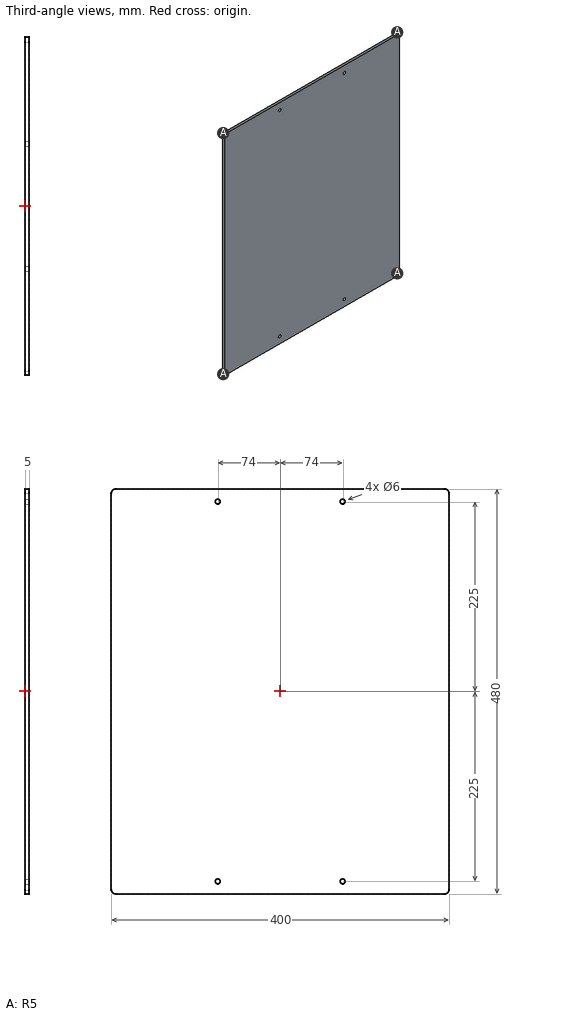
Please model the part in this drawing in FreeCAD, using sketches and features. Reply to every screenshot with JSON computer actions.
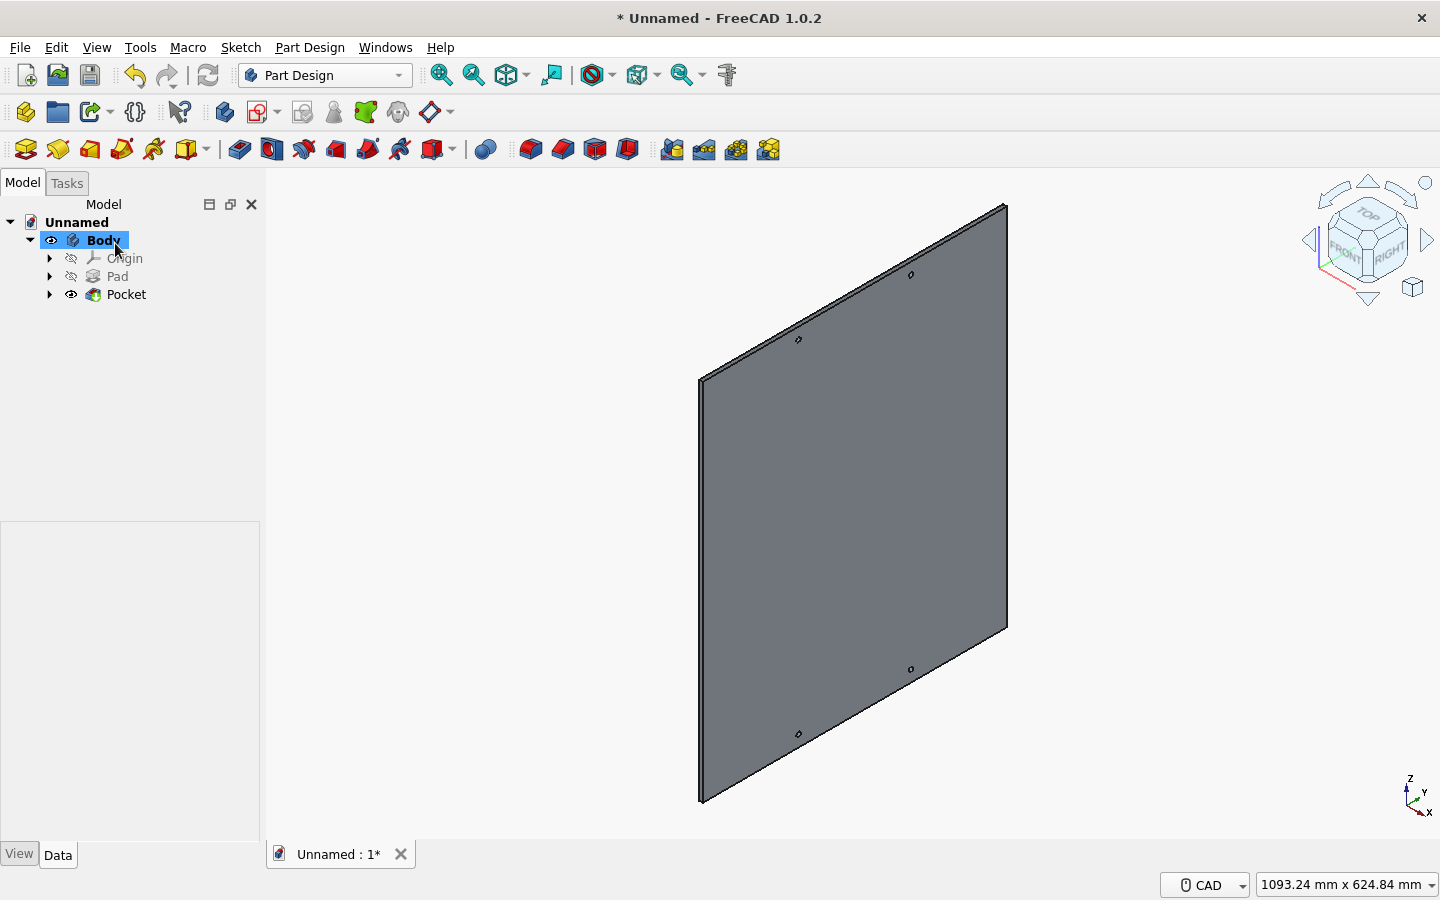
{"action": "scroll", "coordinate": [1005, 204], "scroll_direction": "up", "scroll_amount": 11}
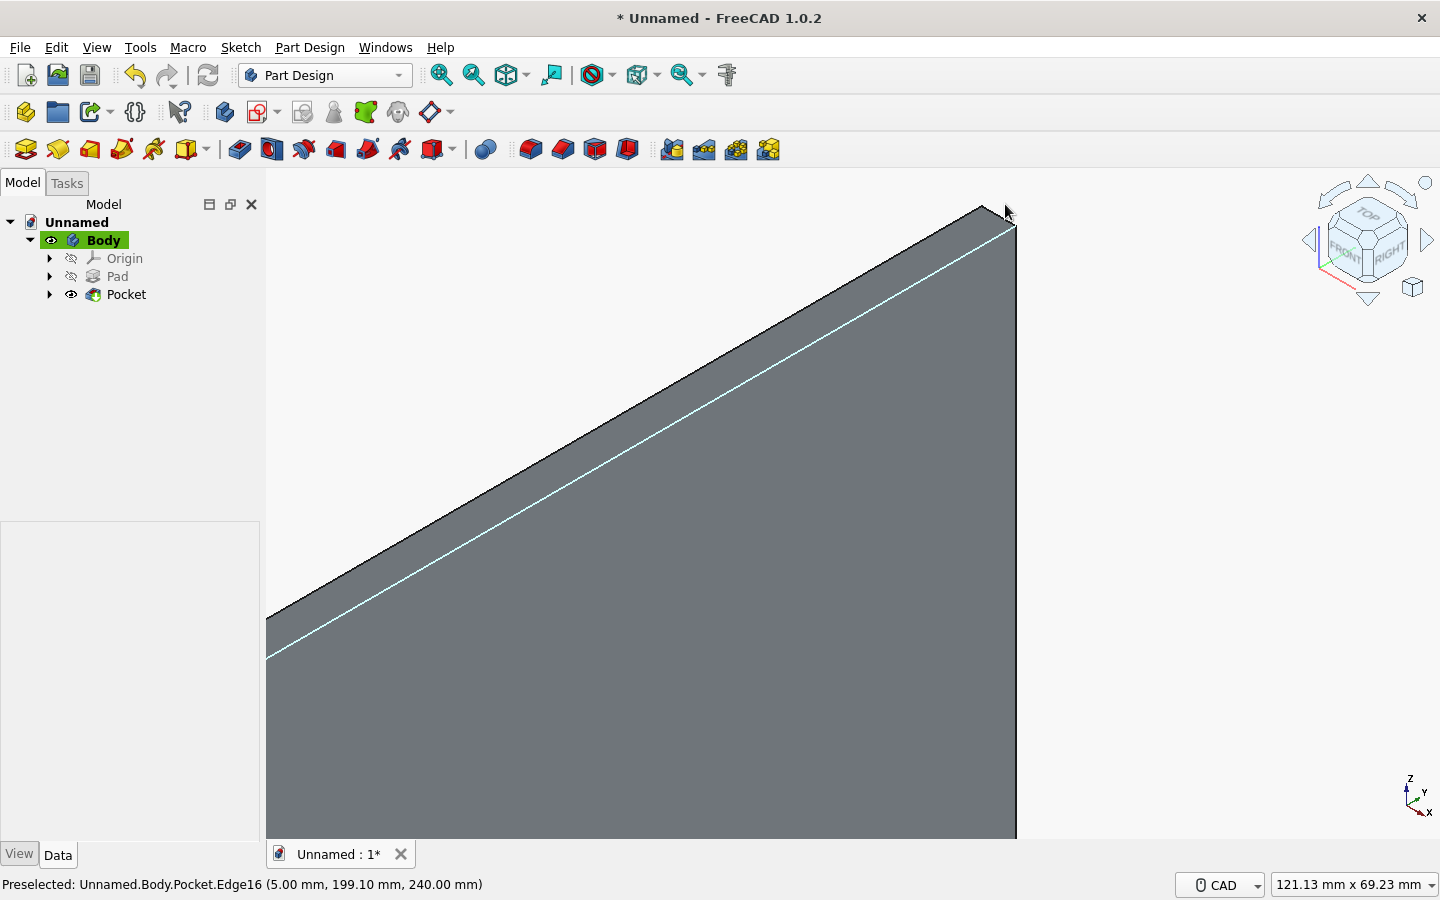
{"action": "left_click", "coordinate": [442, 76]}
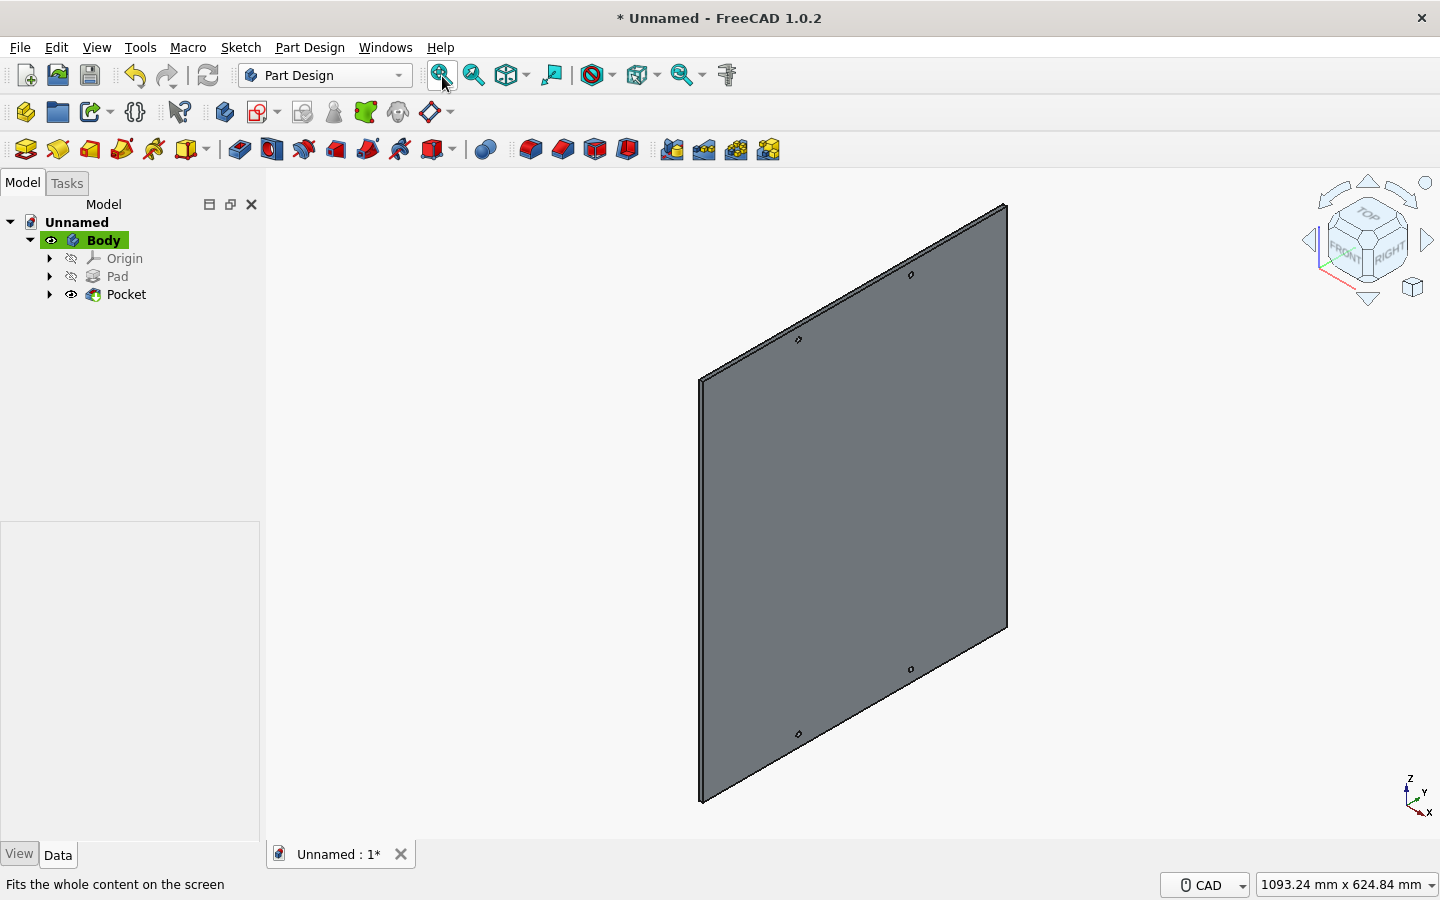
{"action": "key", "text": "2"}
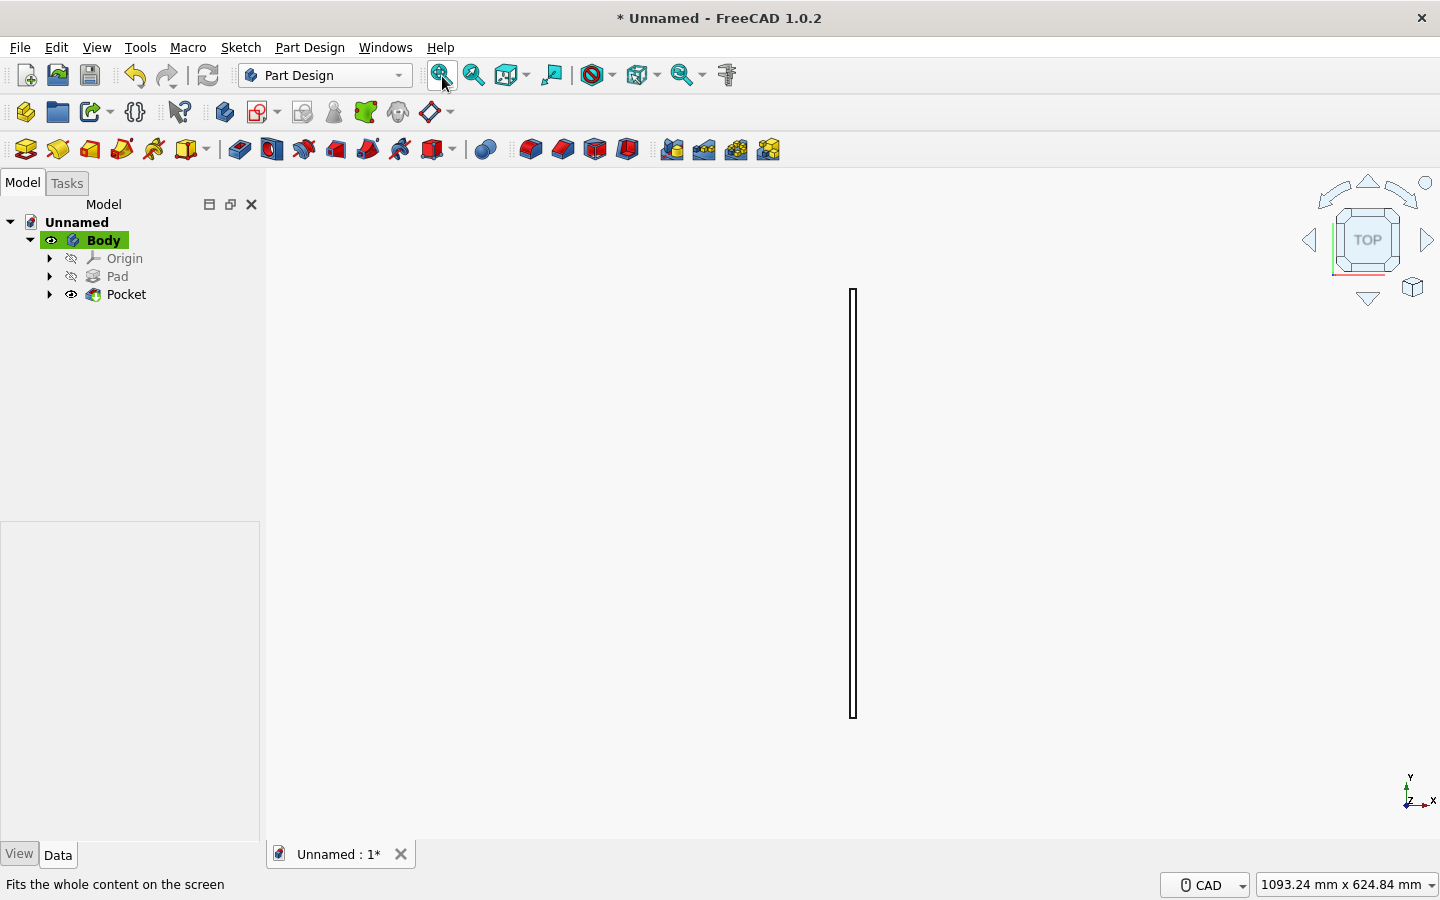
{"action": "scroll", "coordinate": [853, 288], "scroll_direction": "up", "scroll_amount": 11}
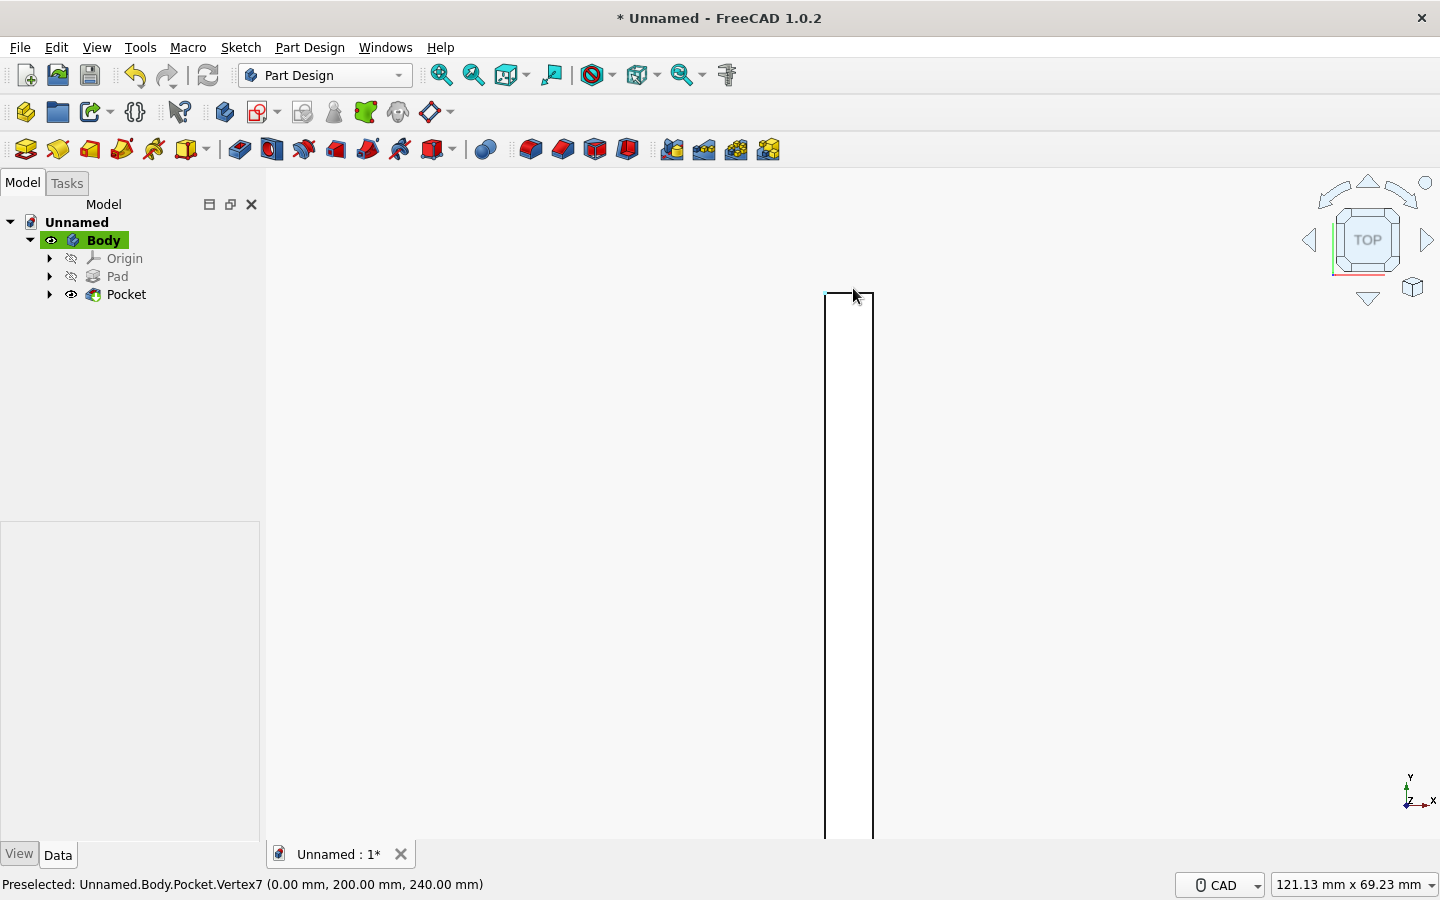
{"action": "left_click", "coordinate": [849, 292]}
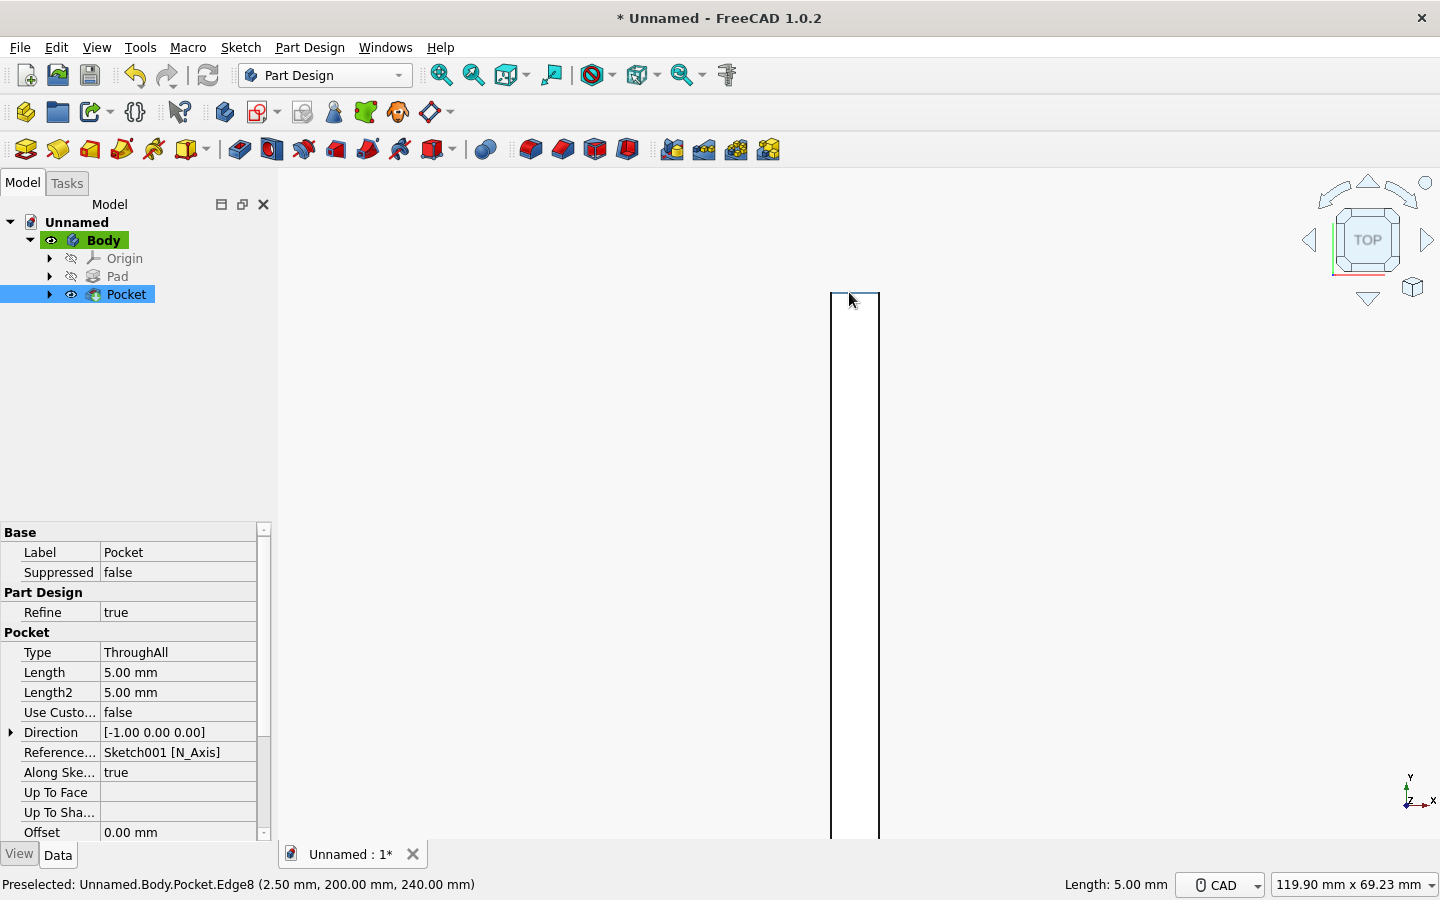
{"action": "key", "text": "v f"}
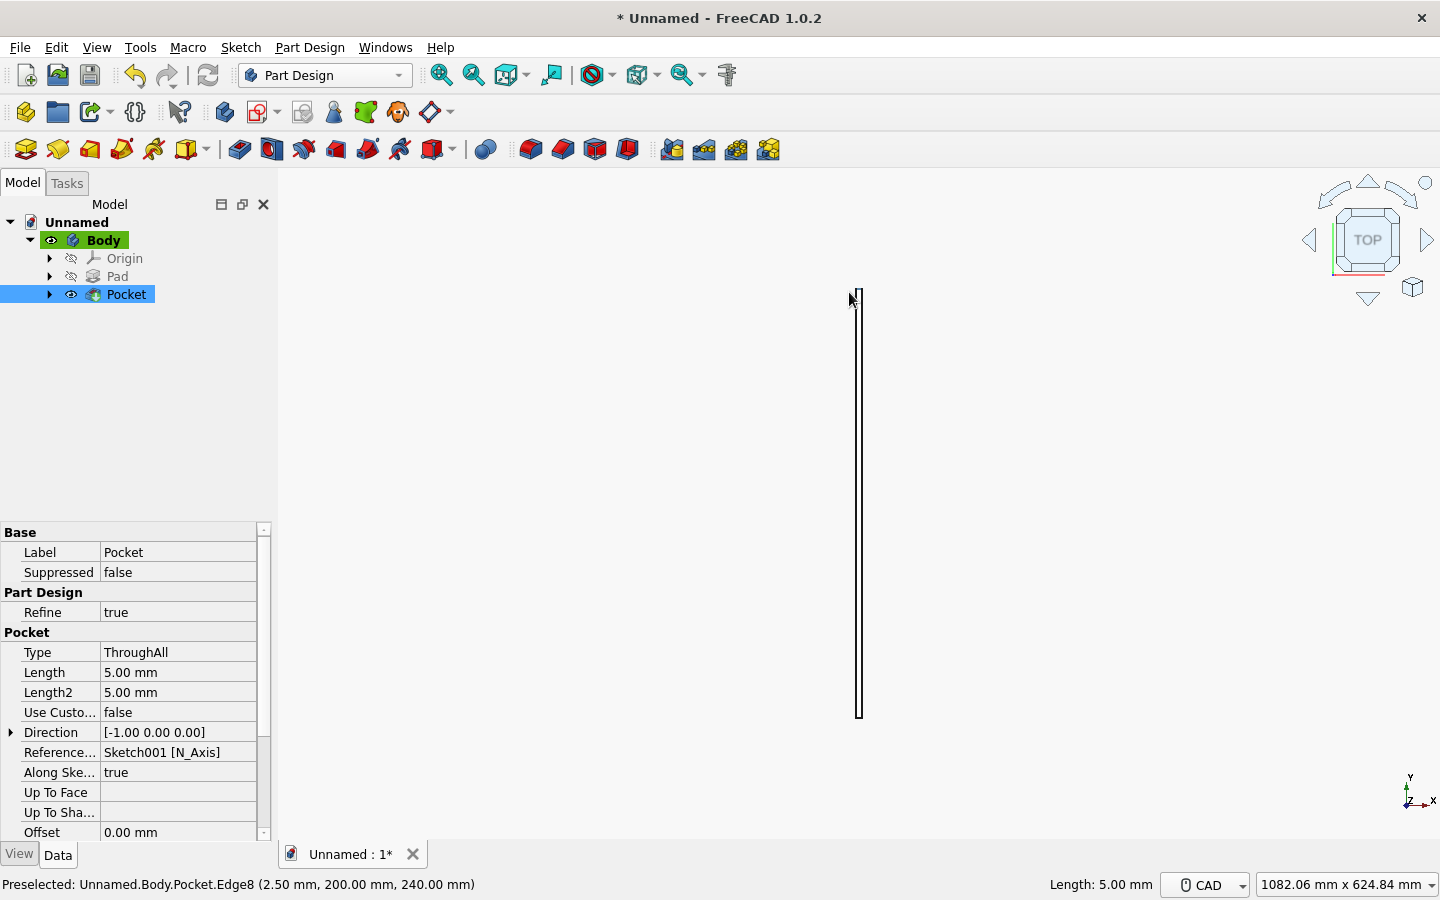
{"action": "key", "text": "1"}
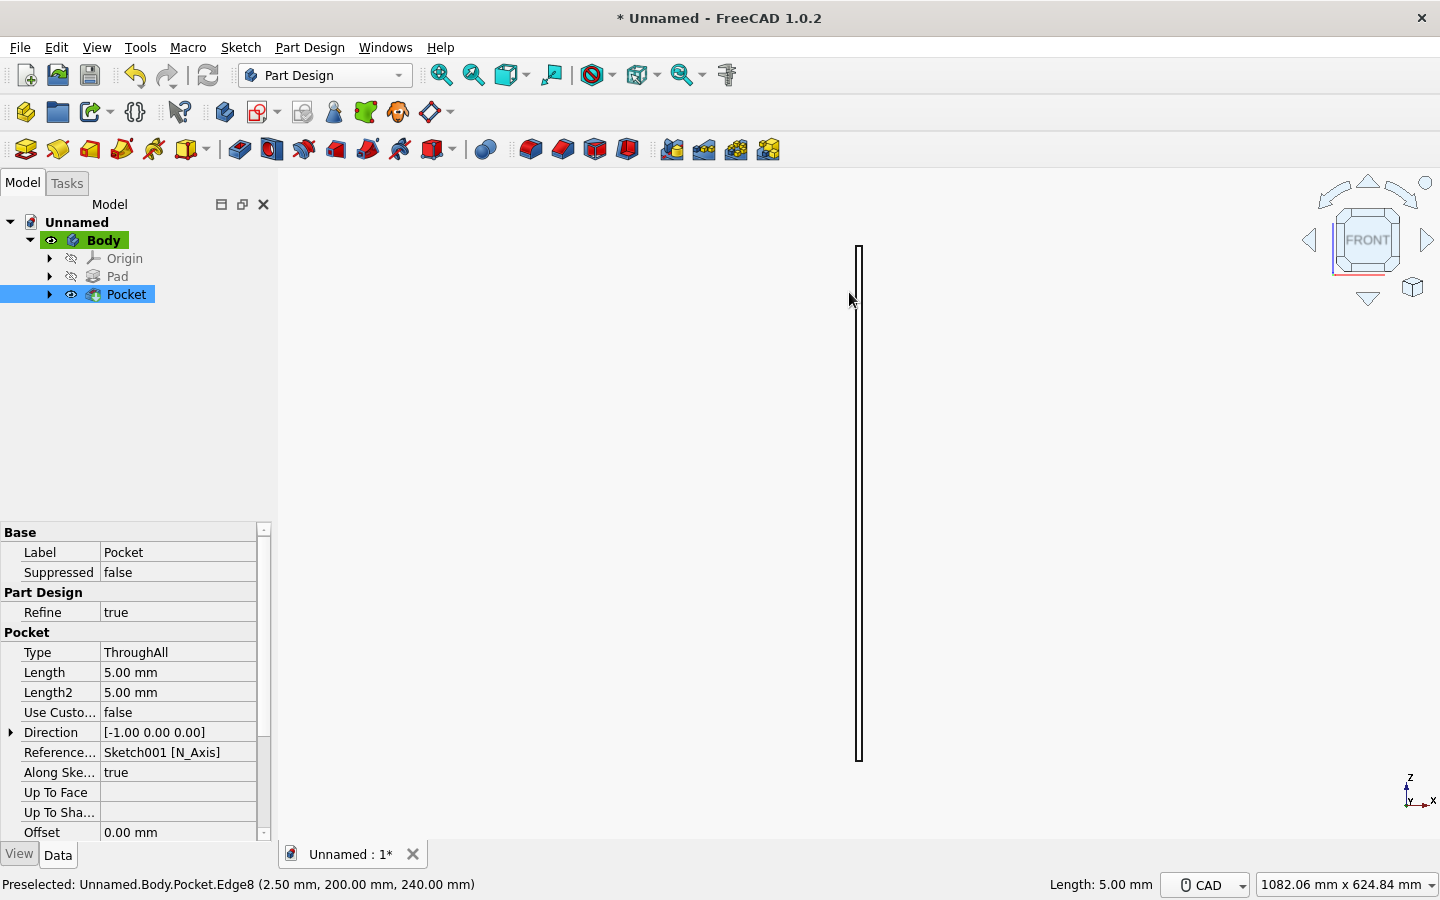
{"action": "scroll", "coordinate": [859, 760], "scroll_direction": "up", "scroll_amount": 11}